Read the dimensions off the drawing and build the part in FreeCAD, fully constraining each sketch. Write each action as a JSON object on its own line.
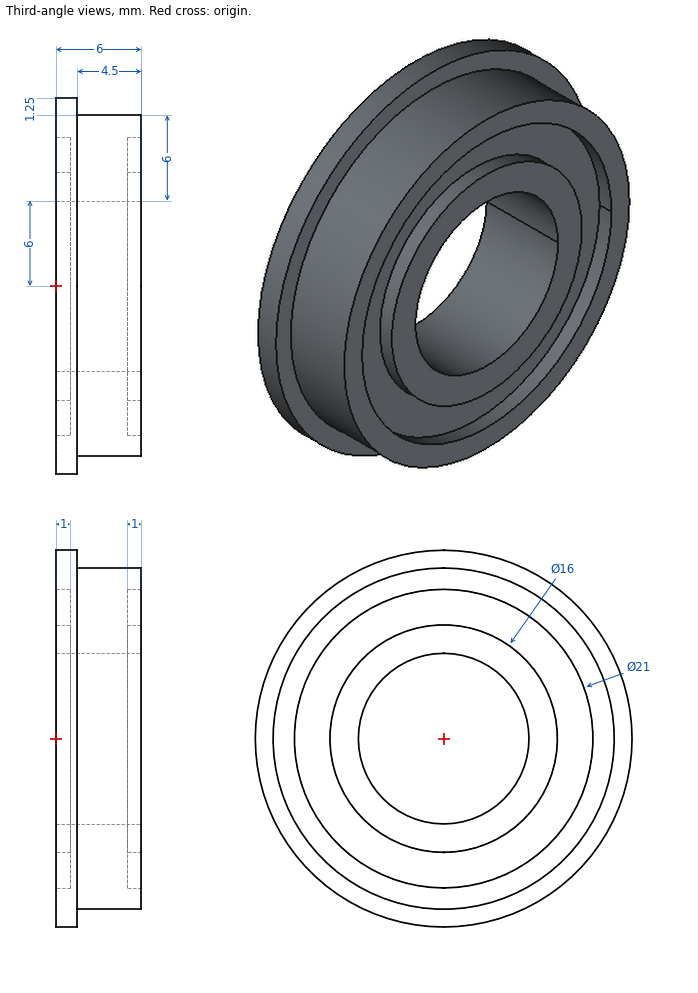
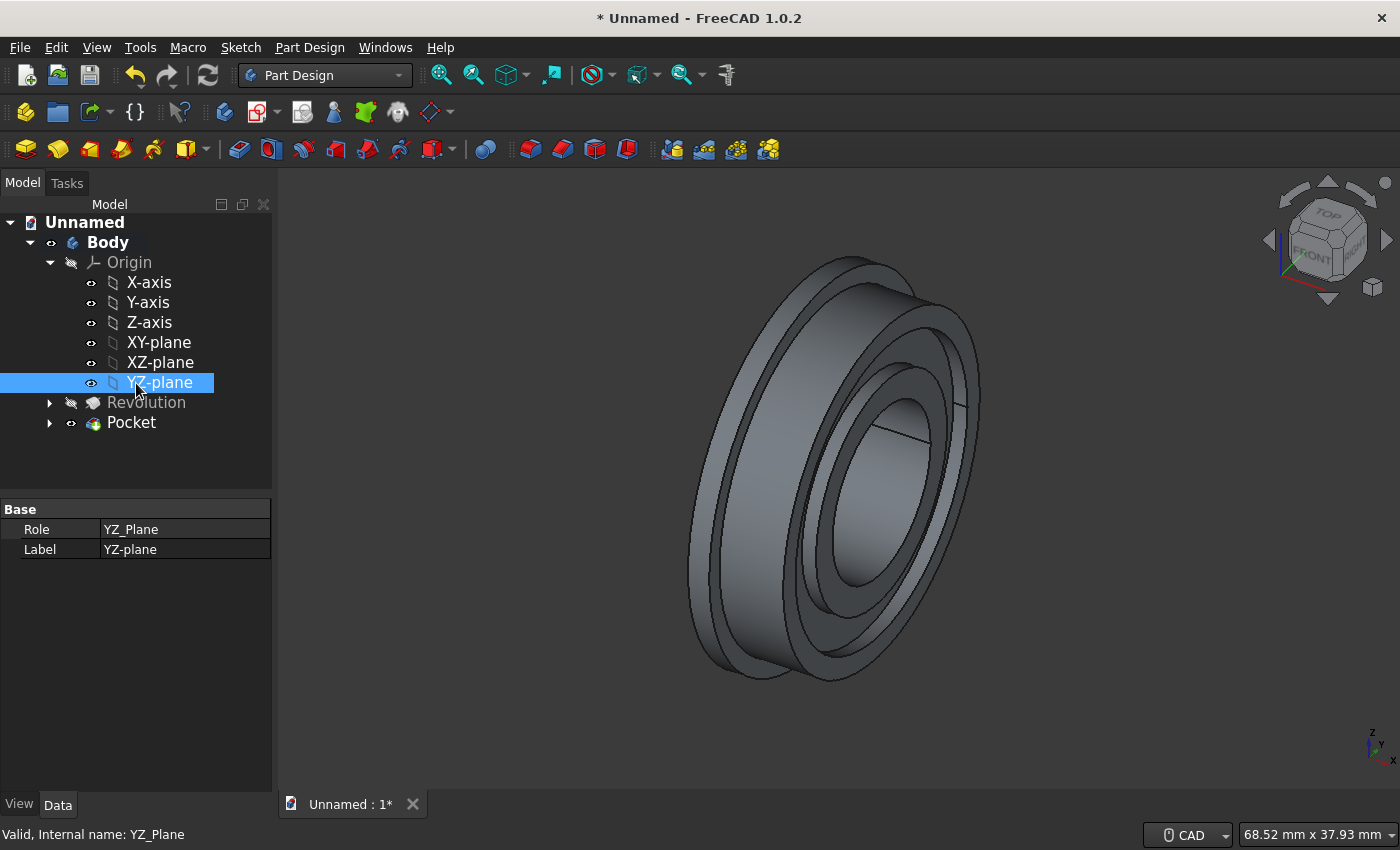
{"action": "left_click", "coordinate": [430, 112]}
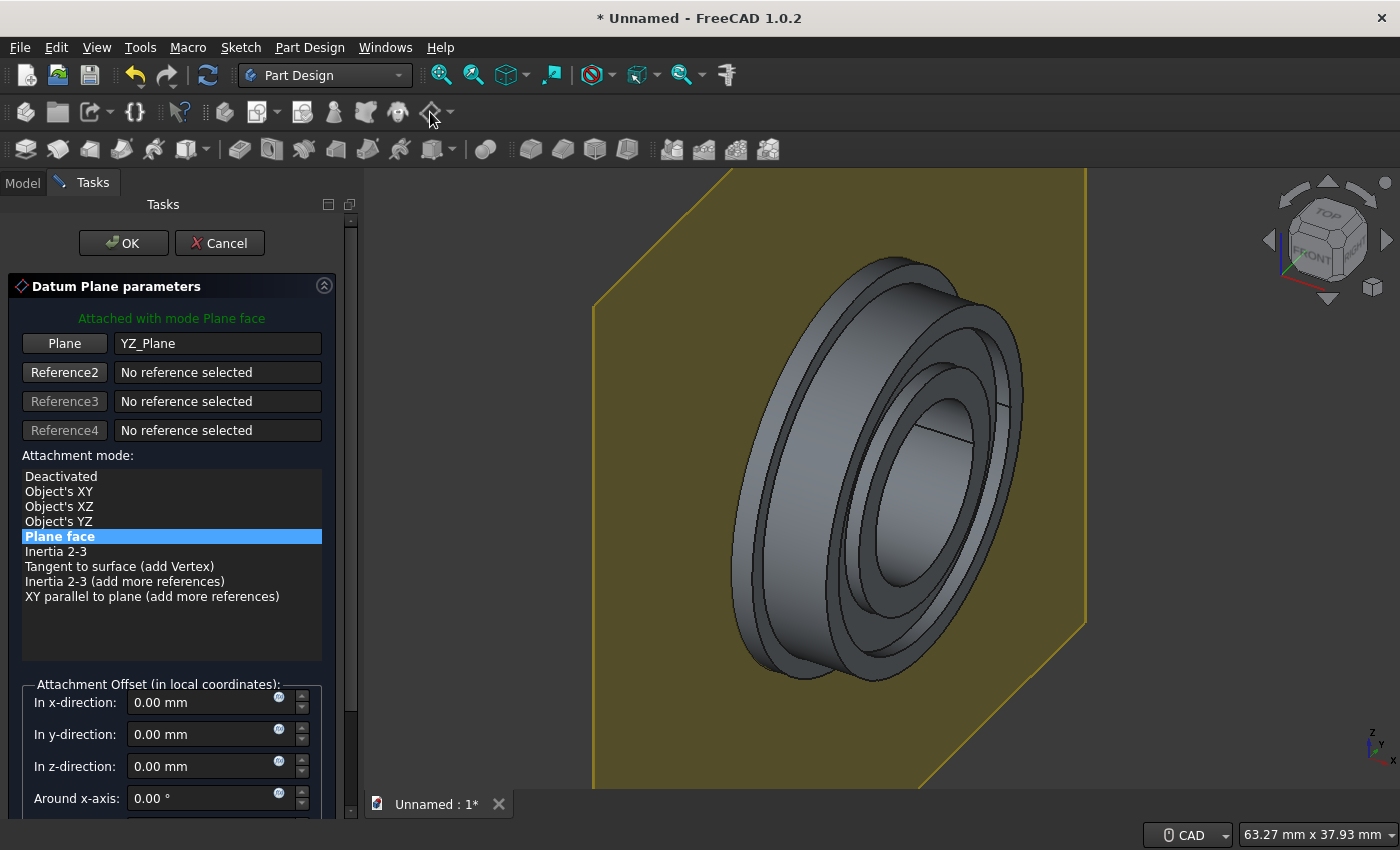
{"action": "triple_click", "coordinate": [210, 766]}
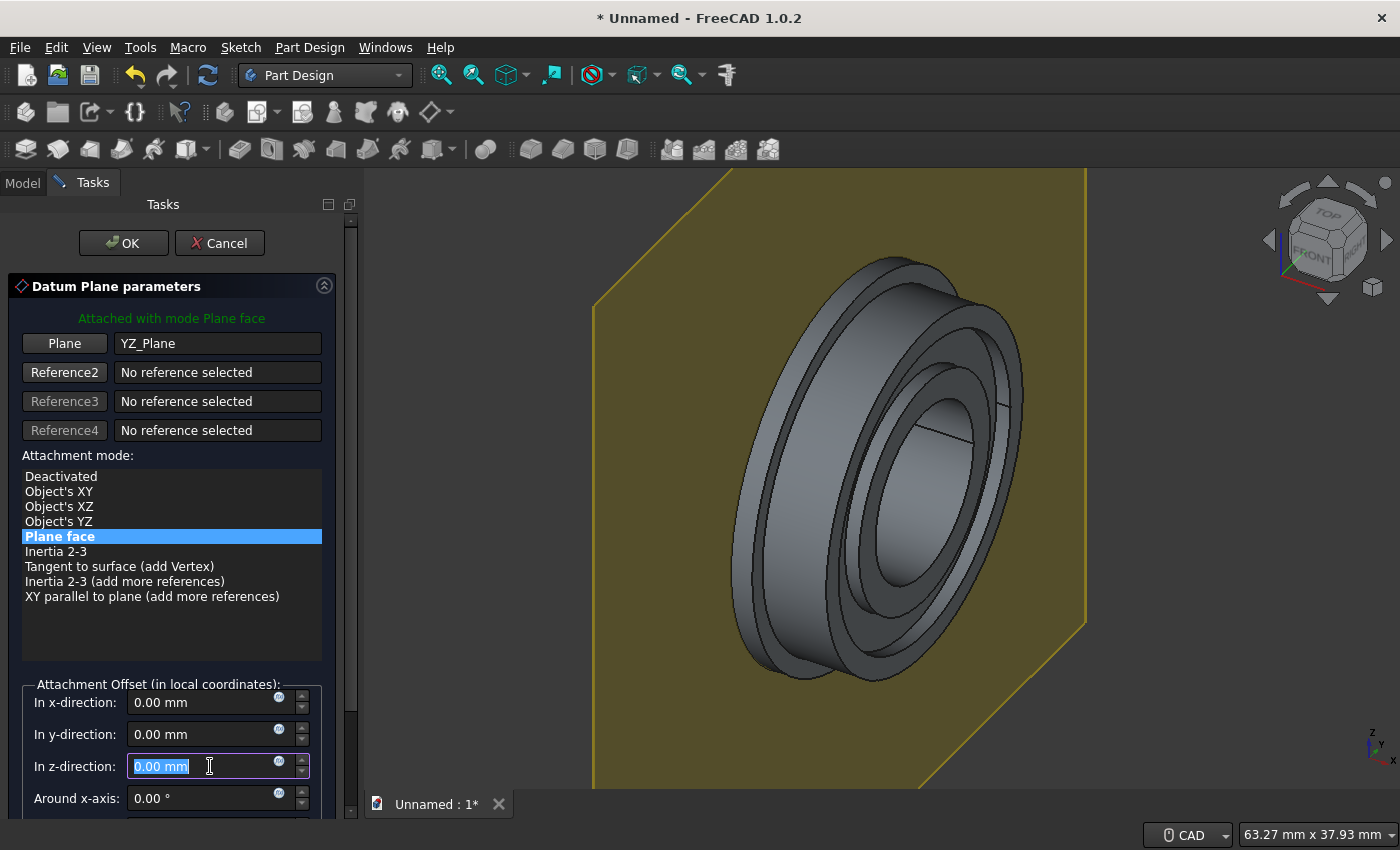
{"action": "type", "text": "1"}
{"action": "key", "text": "Tab"}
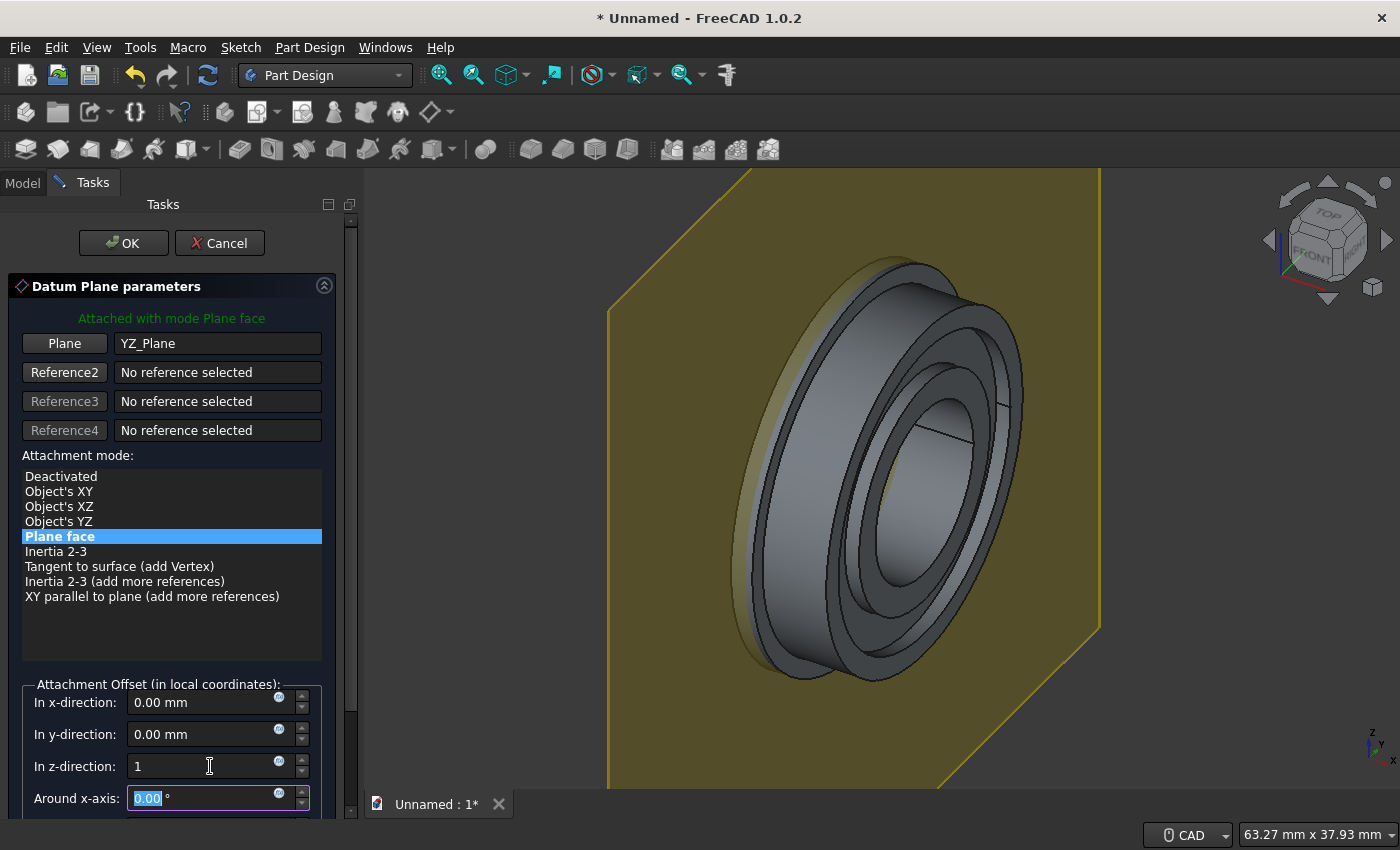
{"action": "left_click", "coordinate": [124, 243]}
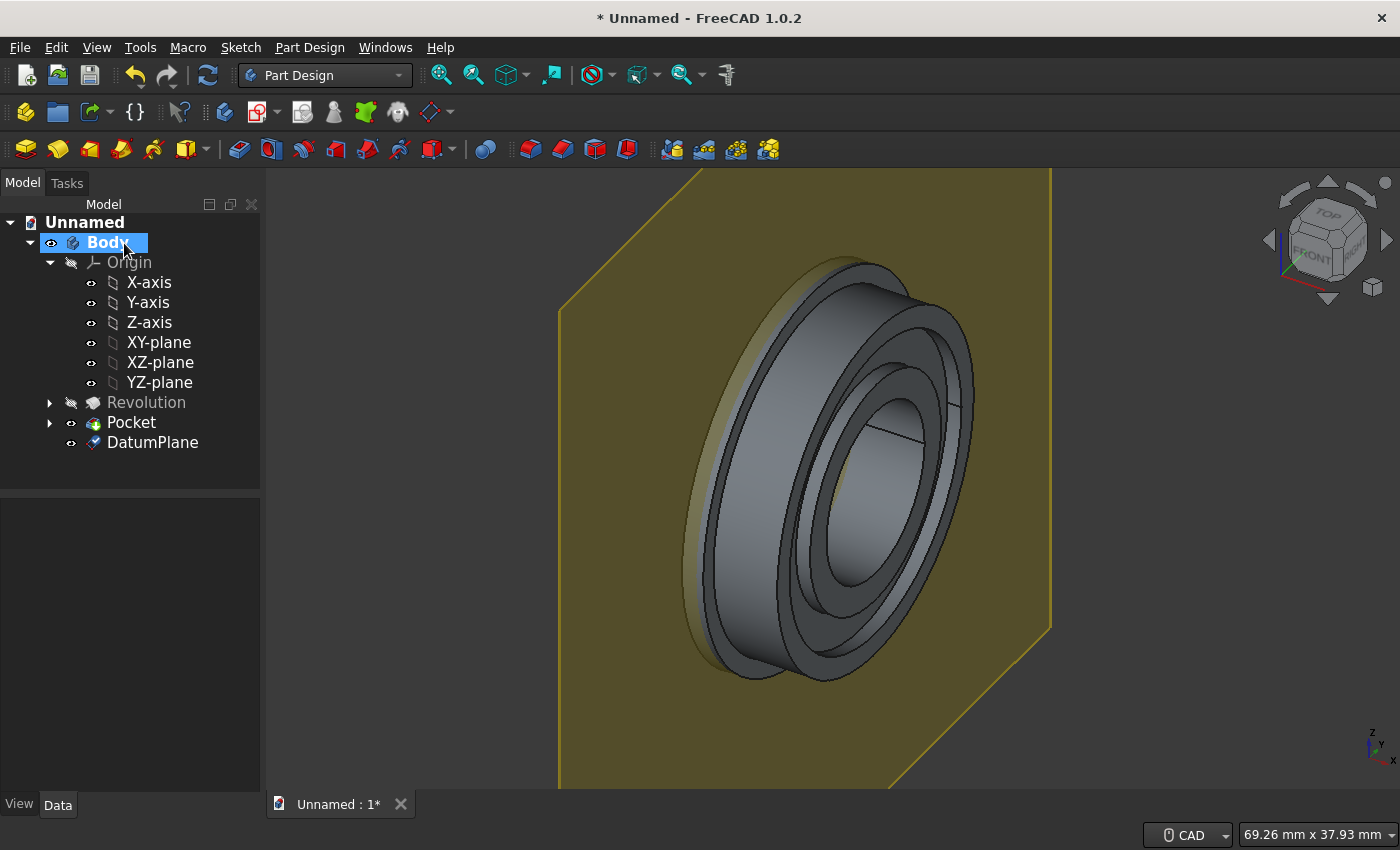
{"action": "left_click", "coordinate": [116, 443]}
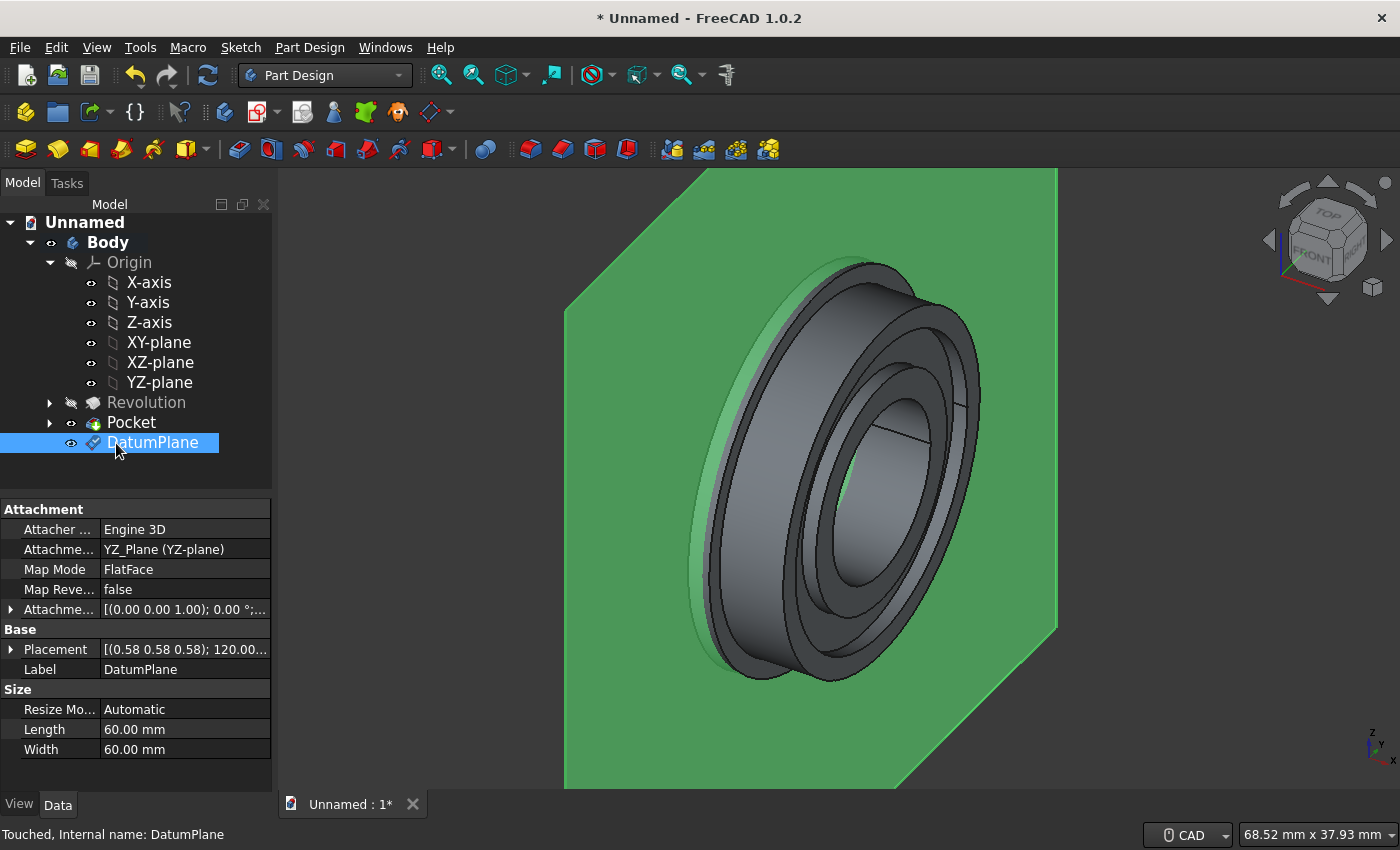
{"action": "left_click", "coordinate": [258, 112]}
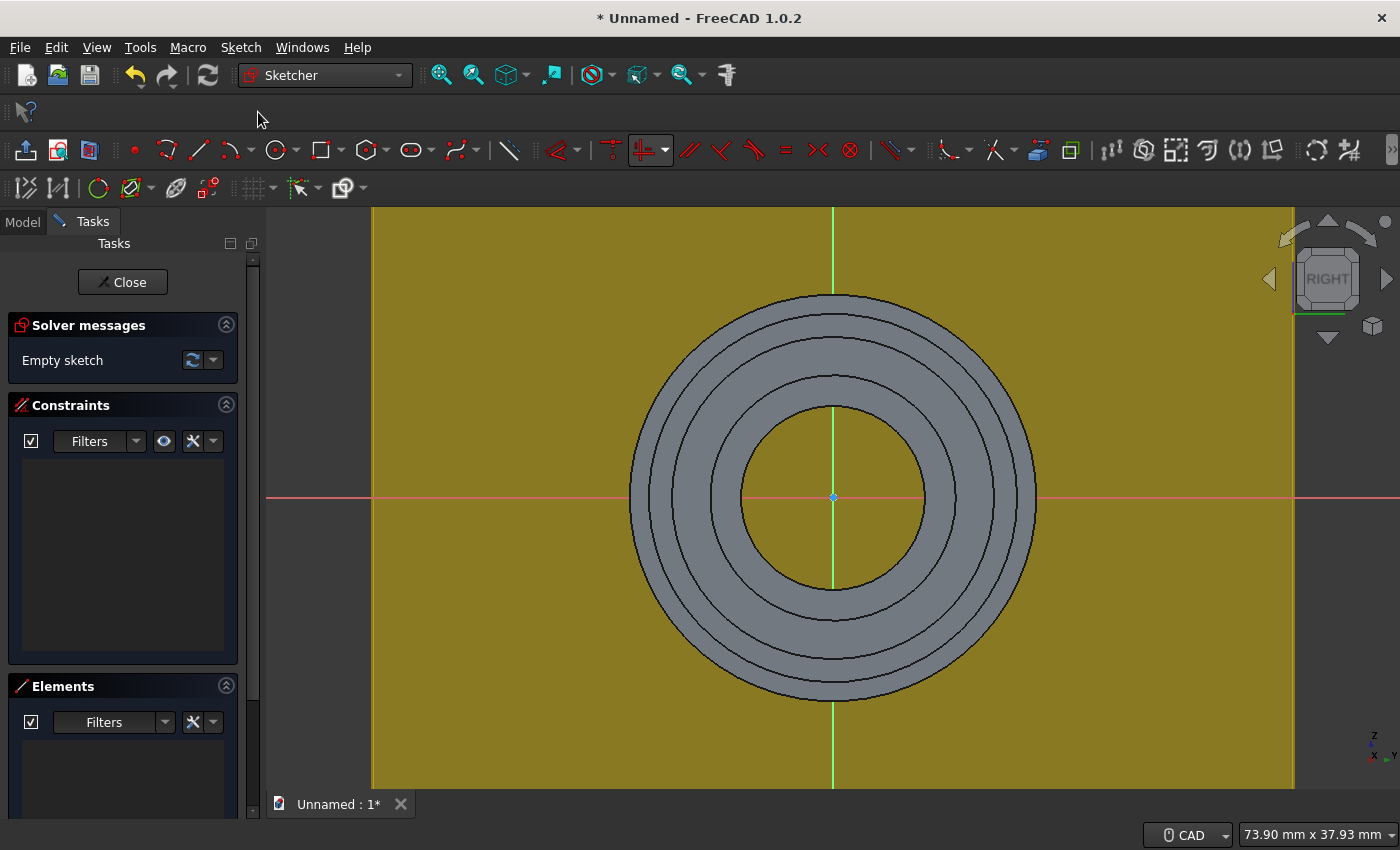
{"action": "left_click", "coordinate": [90, 150]}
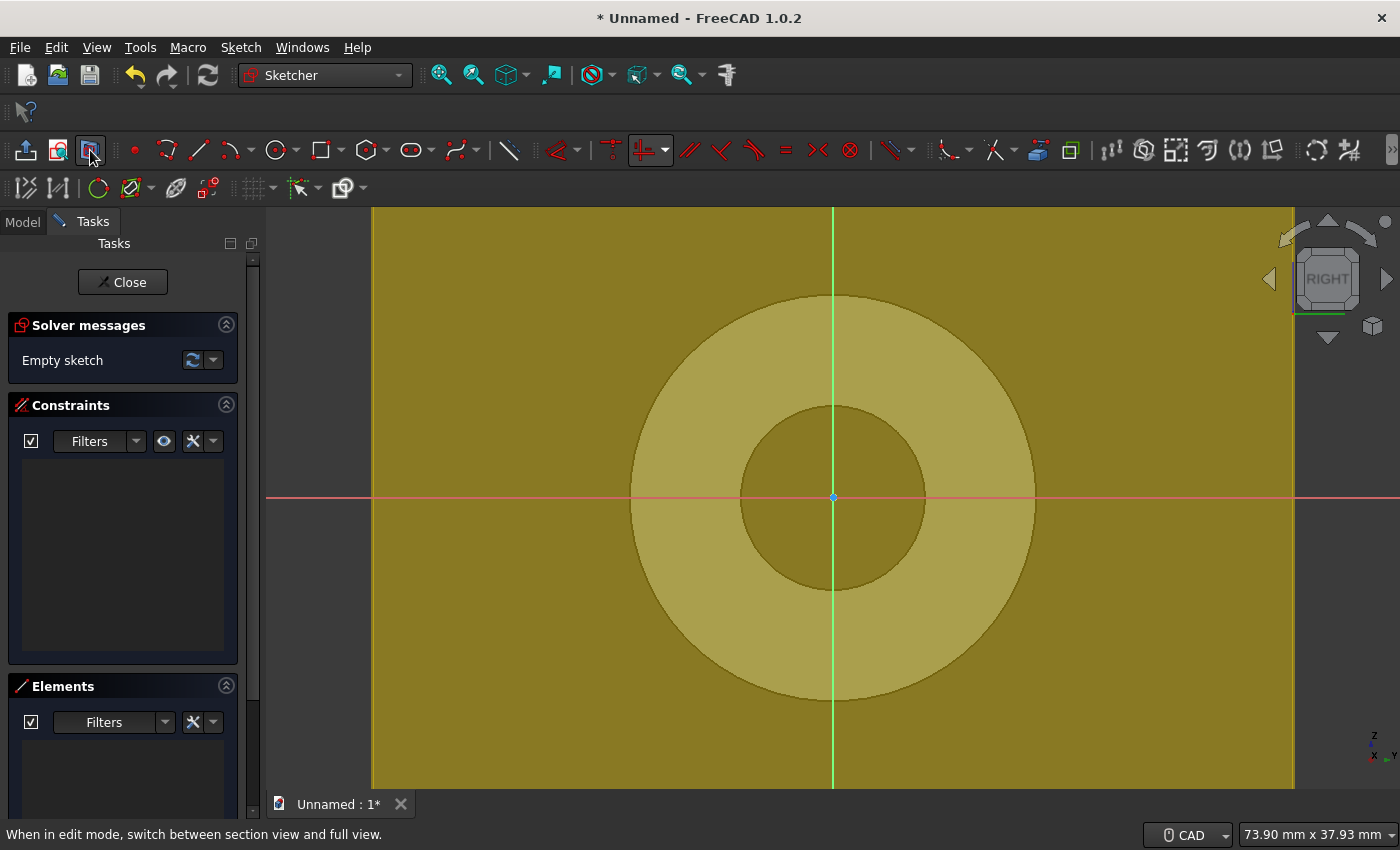
{"action": "left_click", "coordinate": [276, 150]}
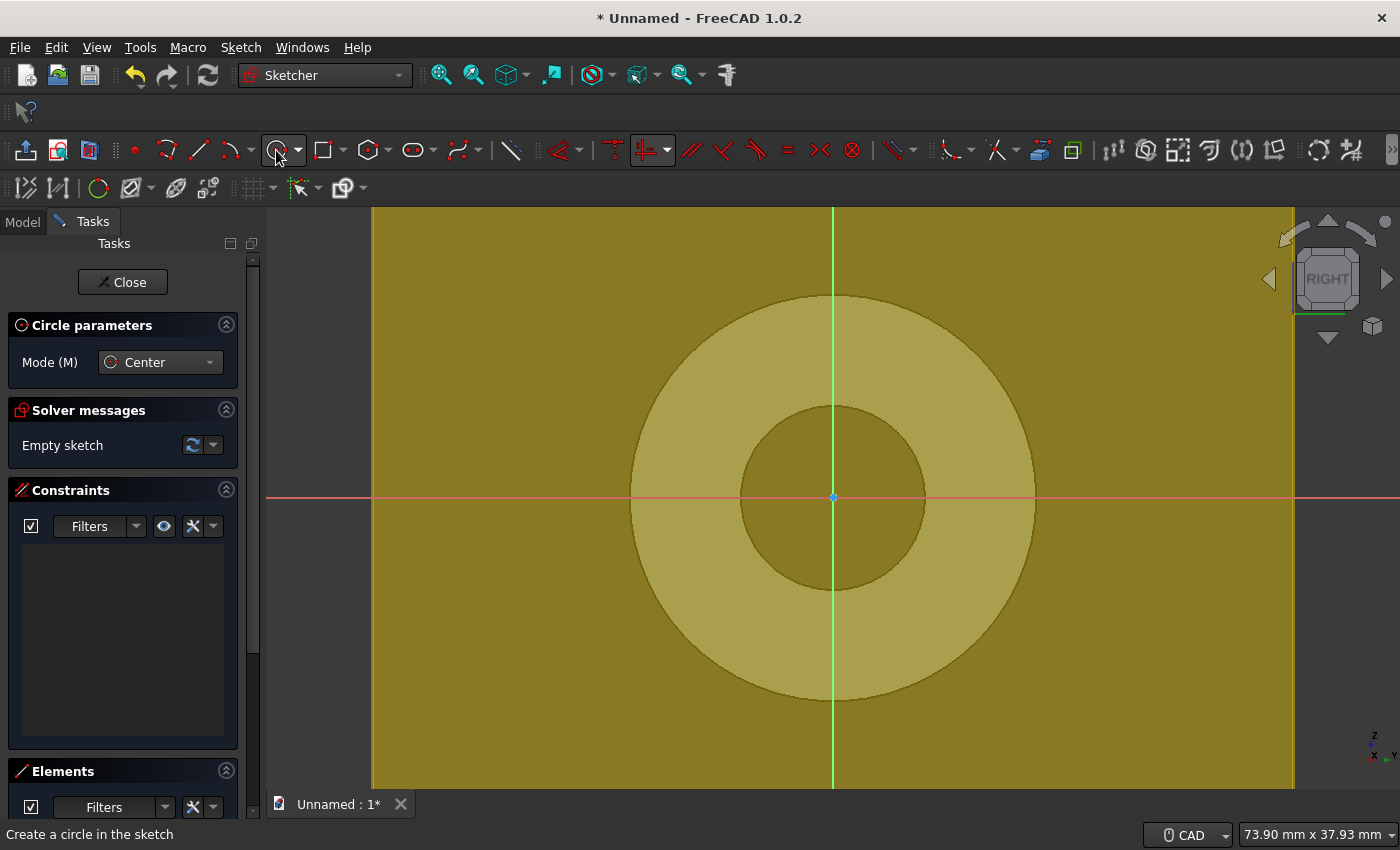
{"action": "left_click", "coordinate": [833, 498]}
{"action": "mouse_move", "coordinate": [947, 384]}